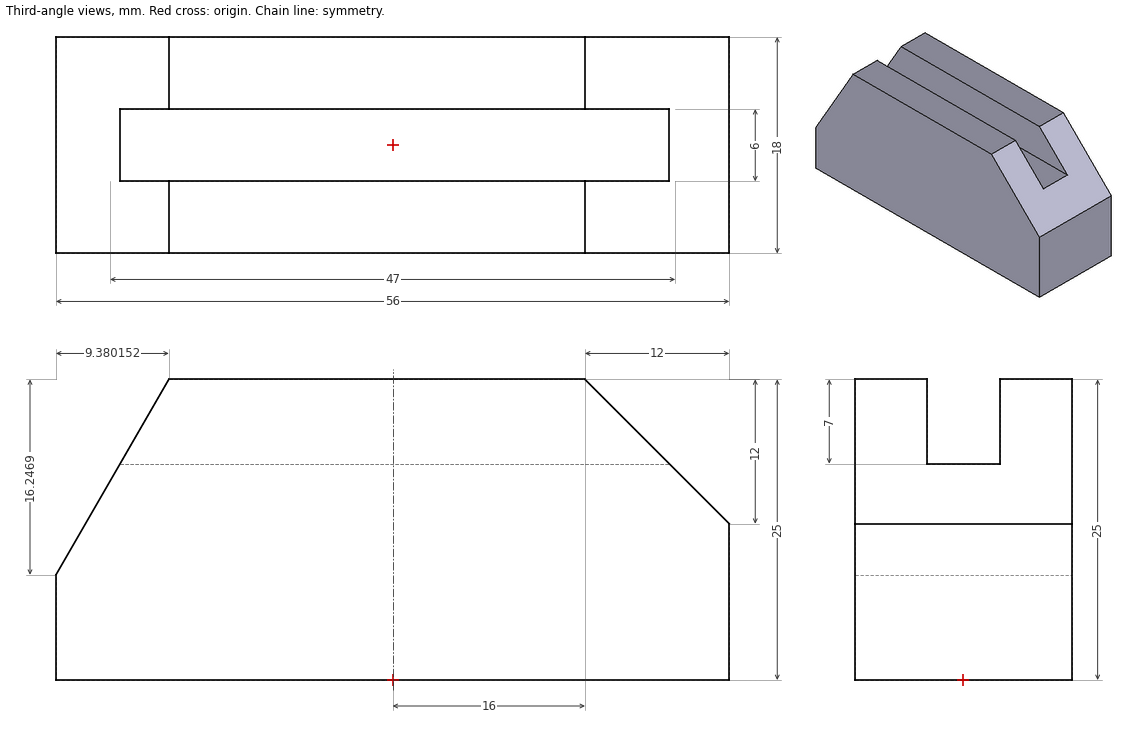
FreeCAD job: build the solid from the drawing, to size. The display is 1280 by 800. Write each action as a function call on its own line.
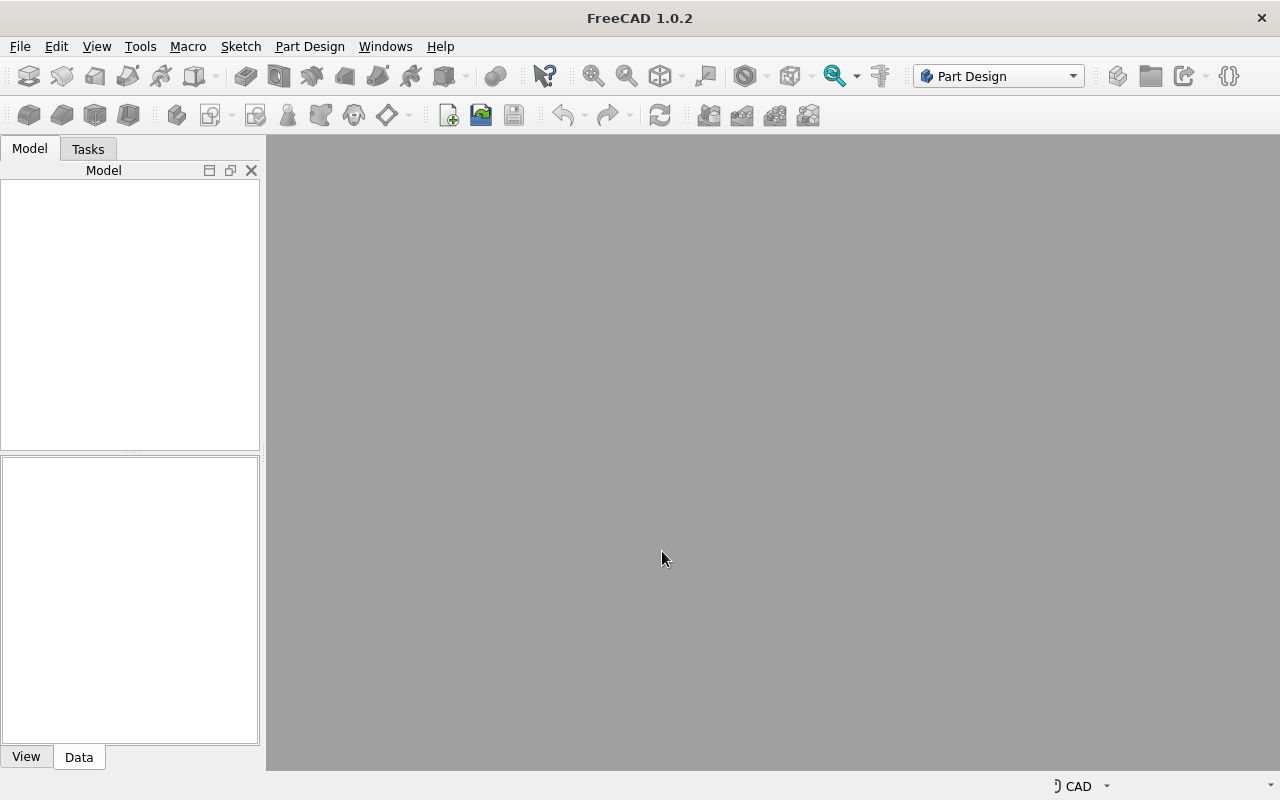
click(448, 116)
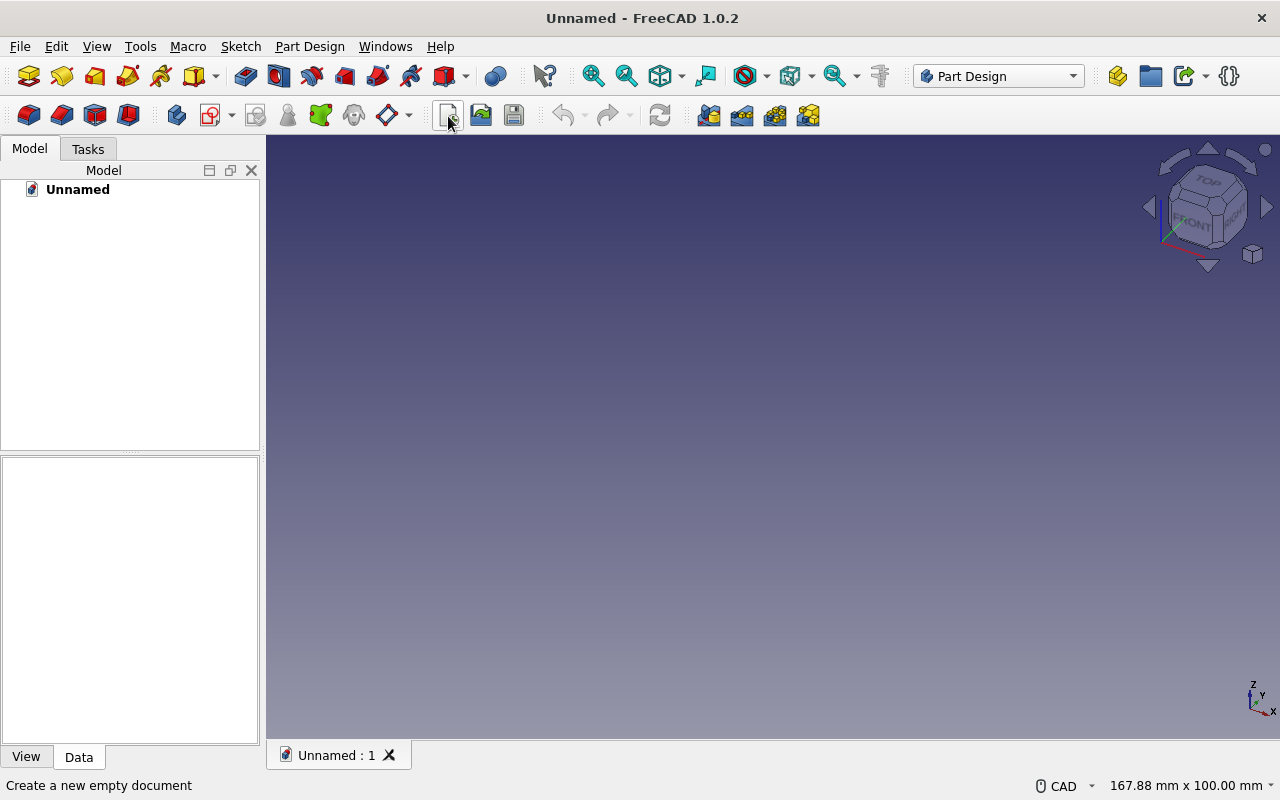
click(210, 116)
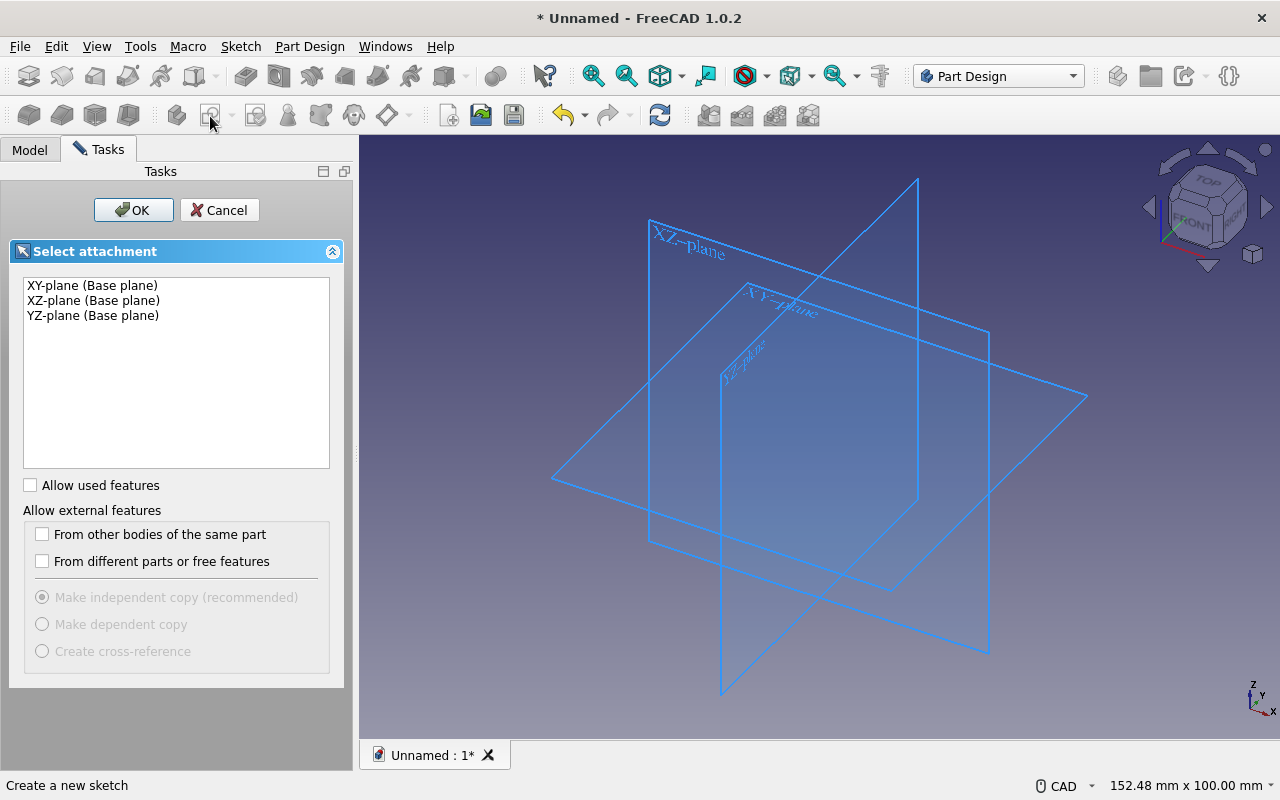
click(84, 286)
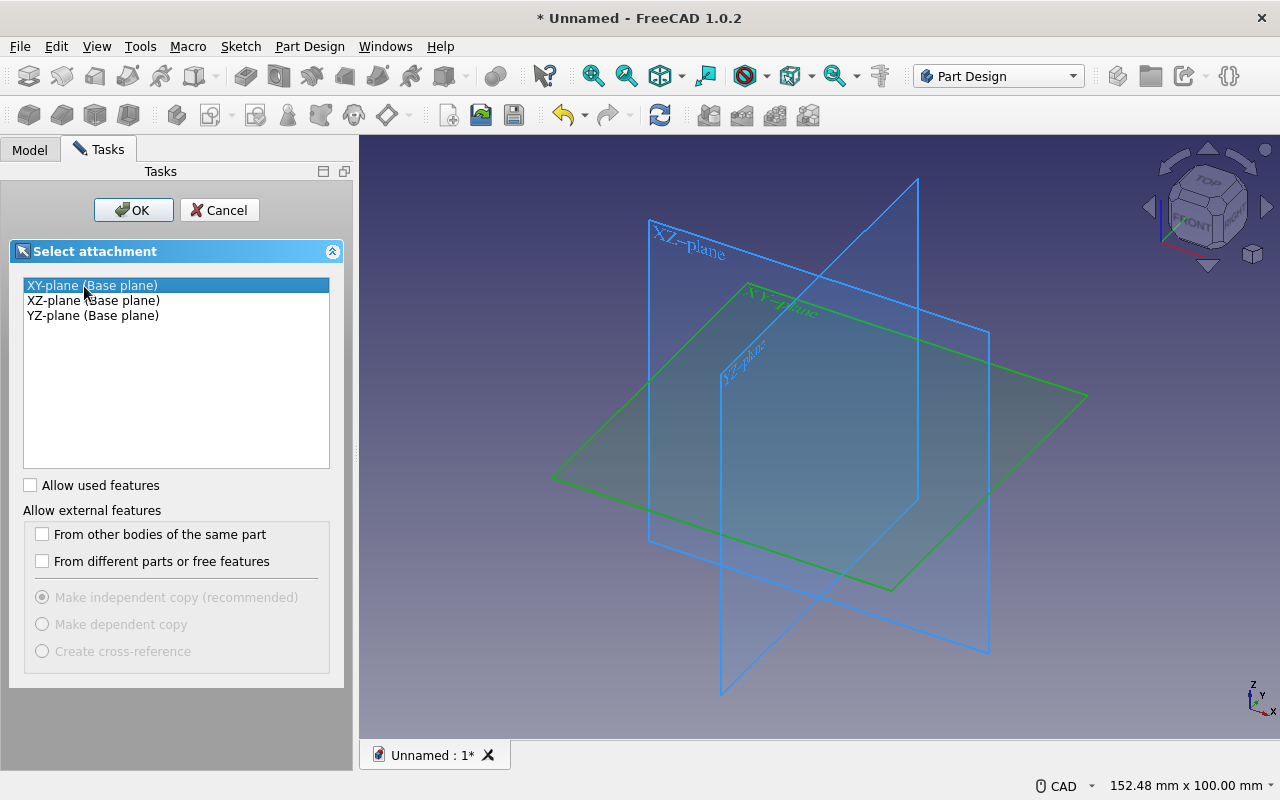
click(134, 210)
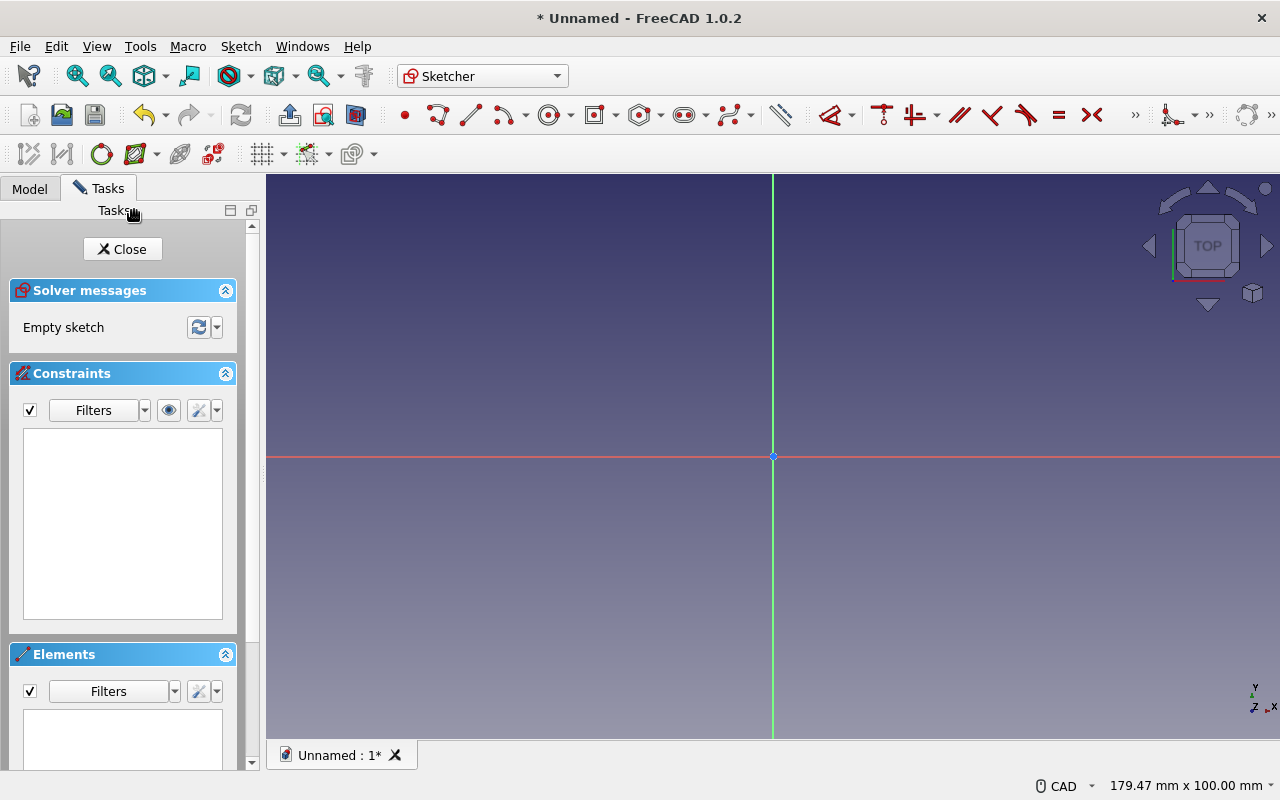
scroll(856, 456, up, 3)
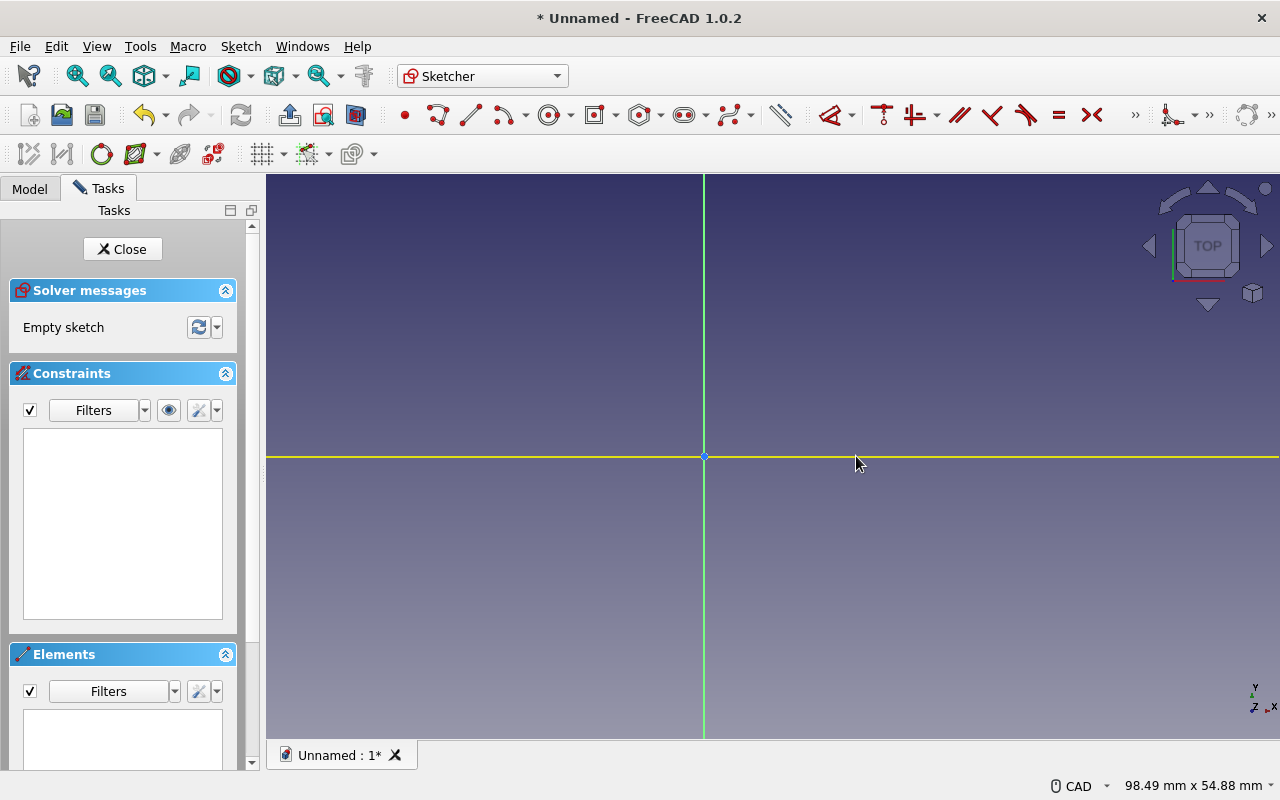
click(594, 116)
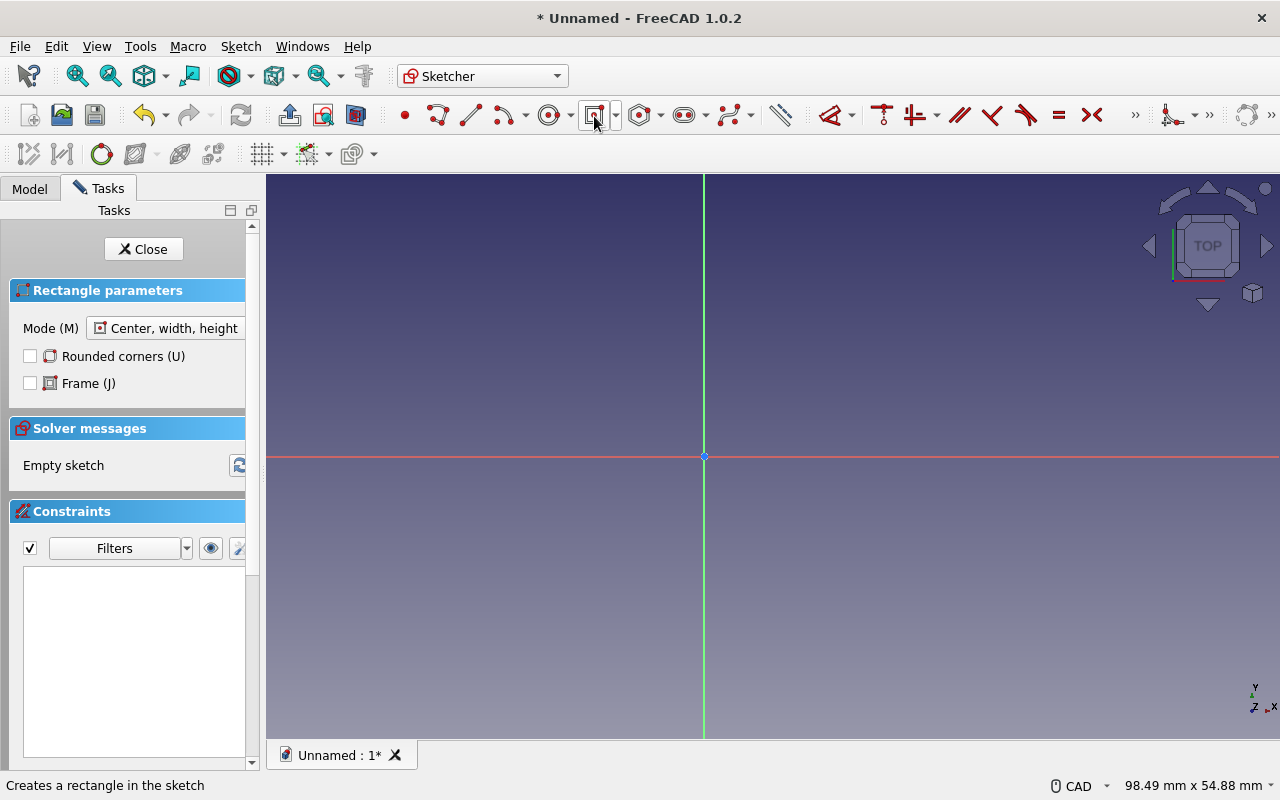
click(704, 456)
move(993, 364)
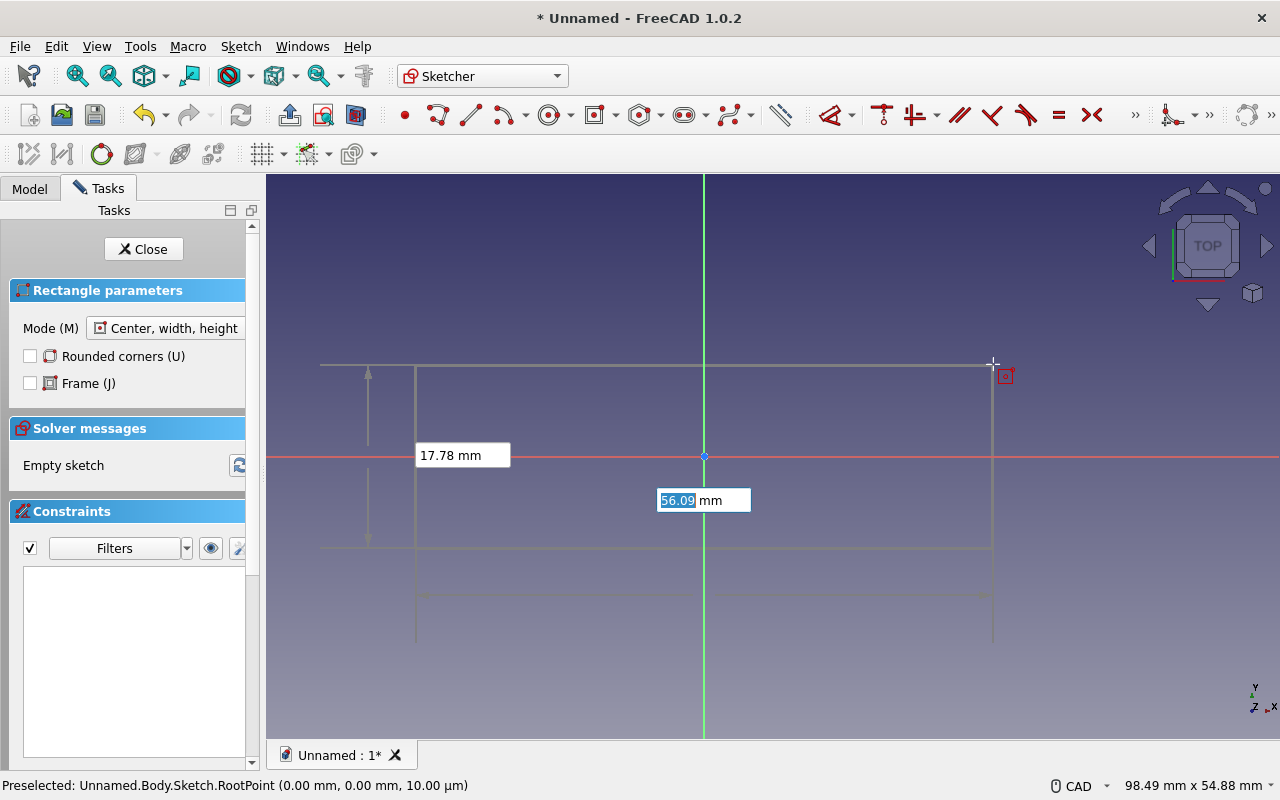
text(56)
key(Tab)
text(18)
key(Return)
key(Escape)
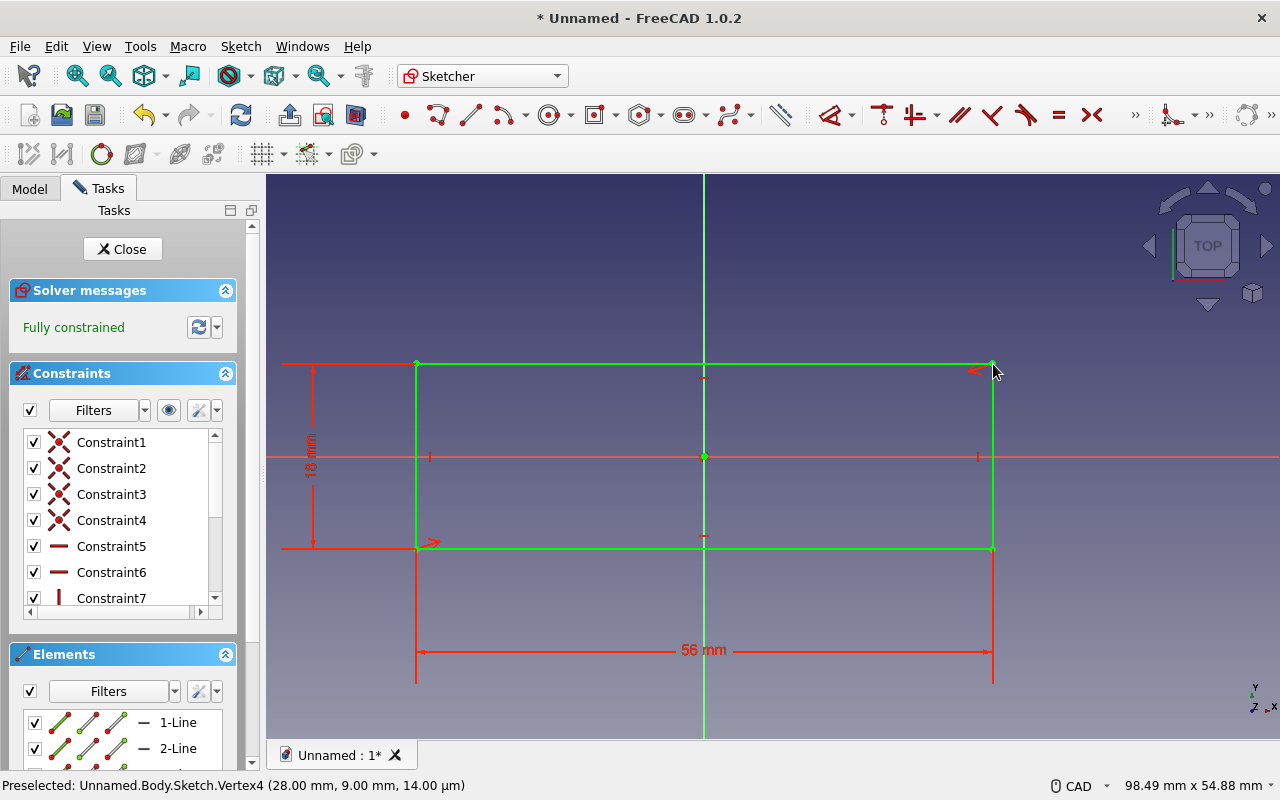
click(123, 249)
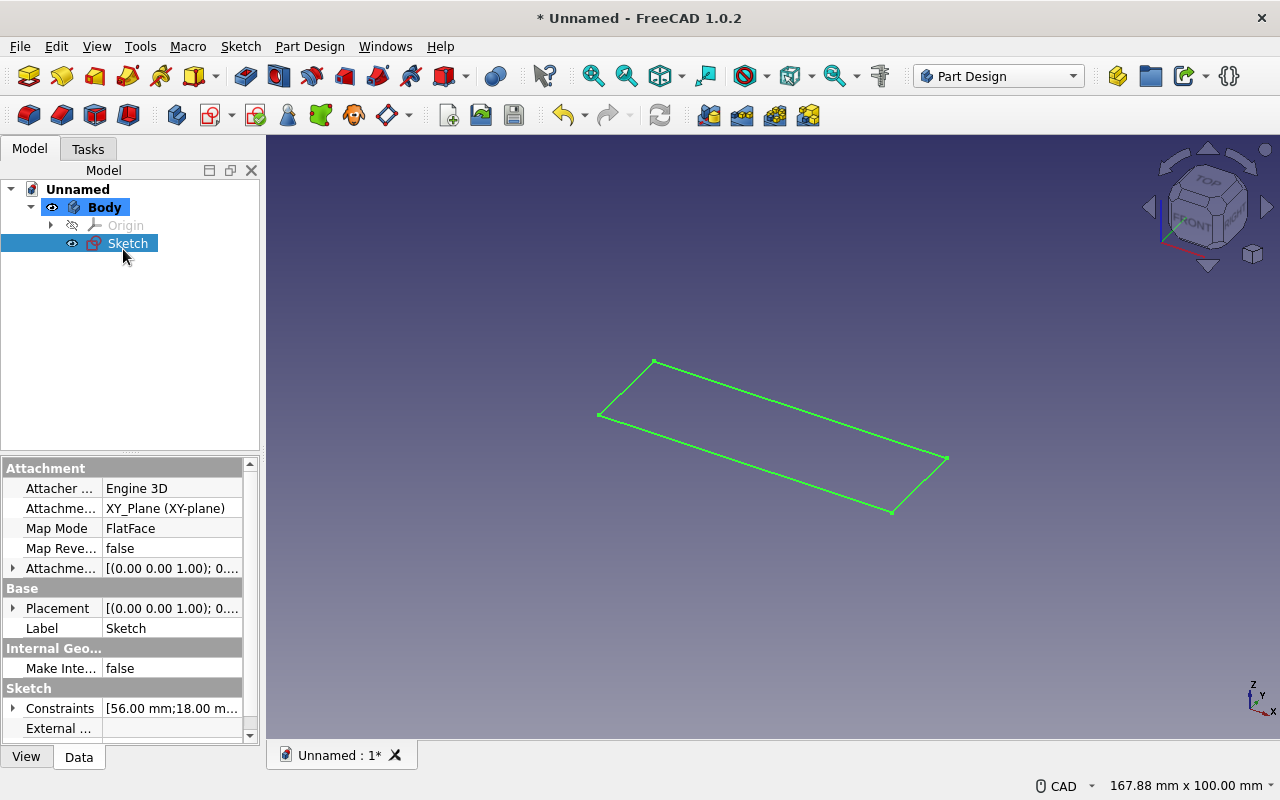
click(29, 76)